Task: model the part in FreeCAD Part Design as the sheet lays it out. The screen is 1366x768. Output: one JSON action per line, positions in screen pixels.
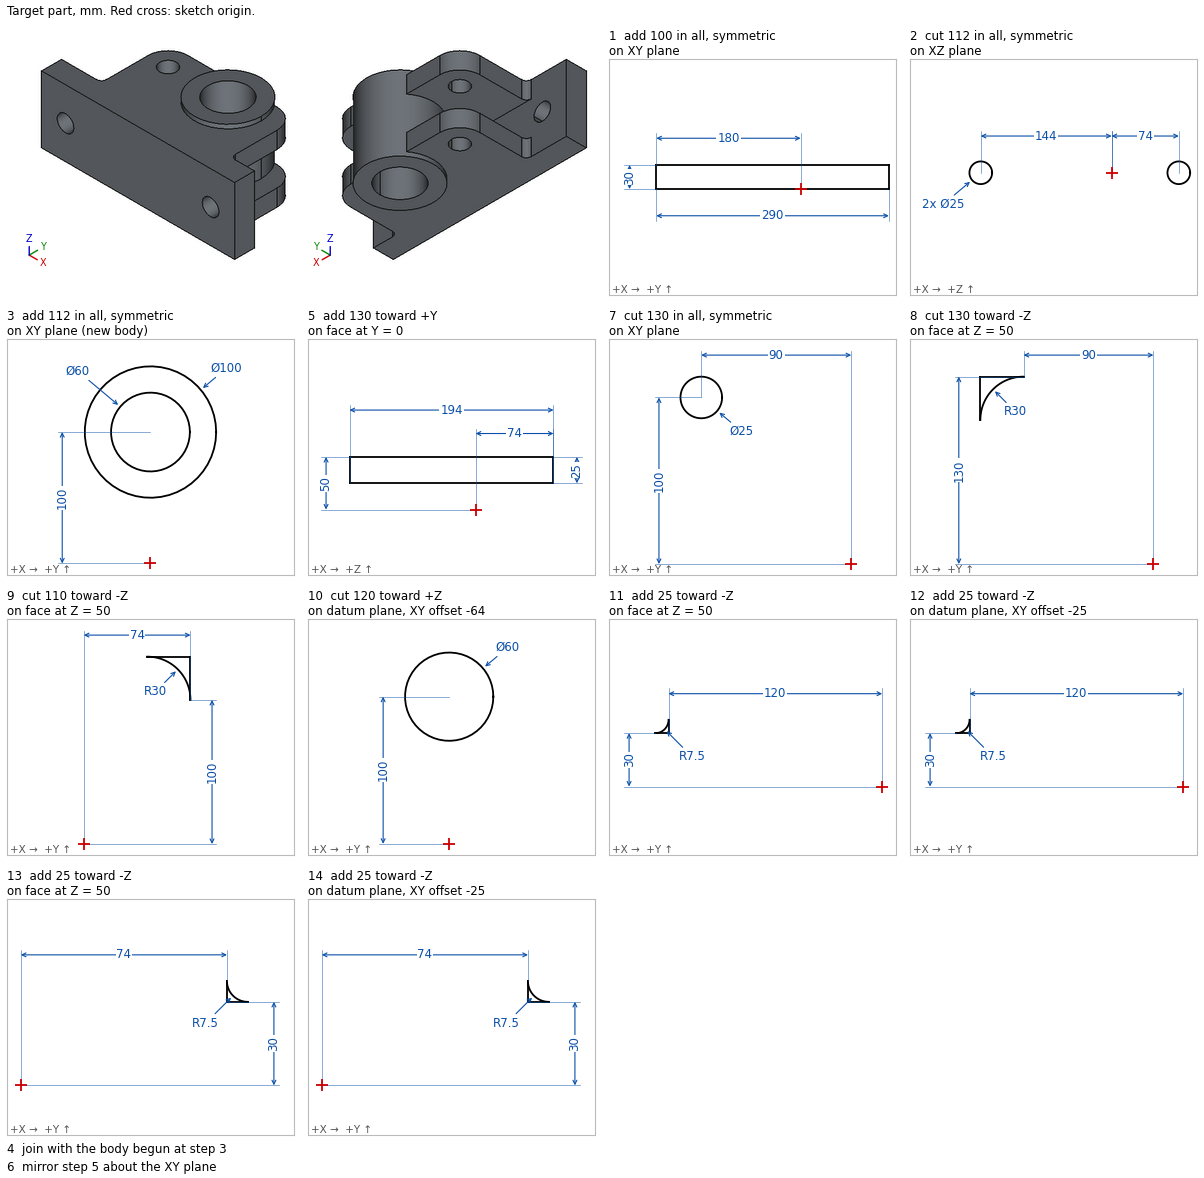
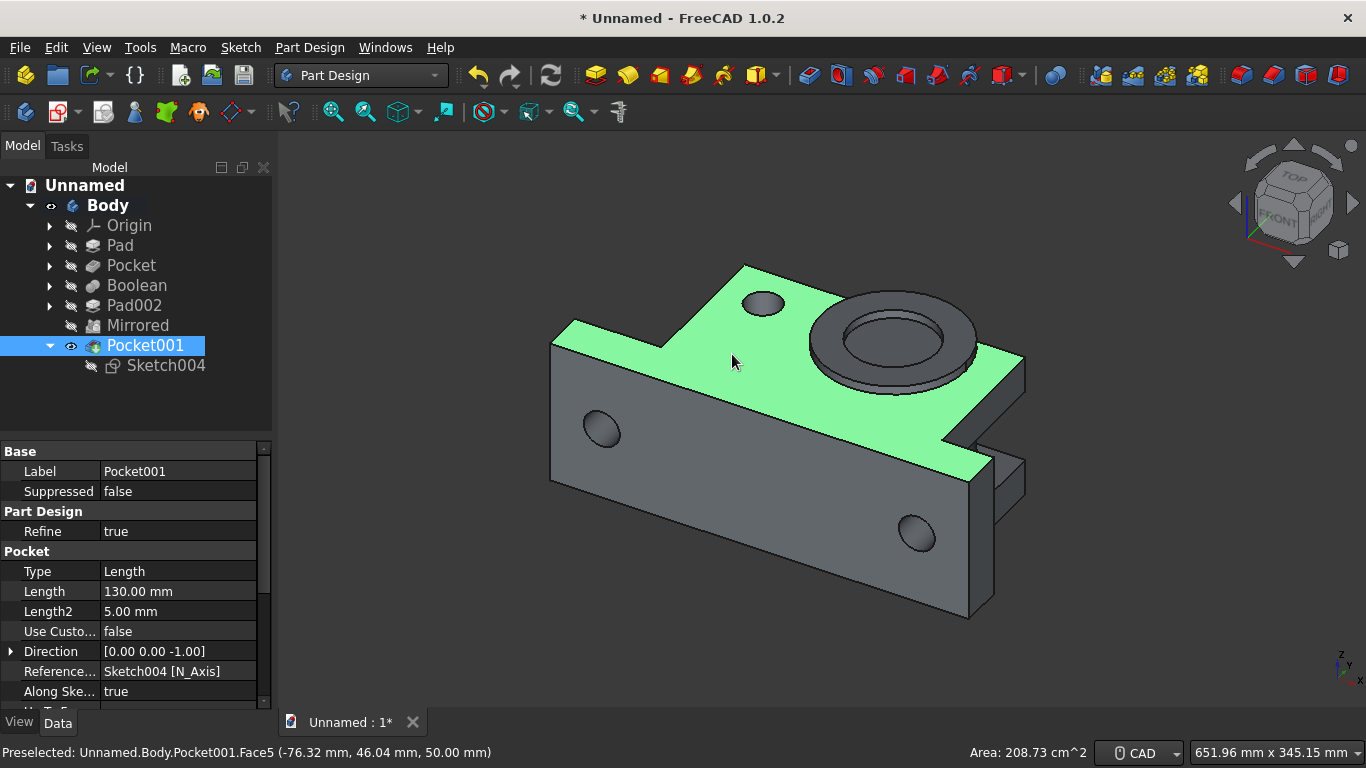
{"action": "left_click", "coordinate": [58, 112]}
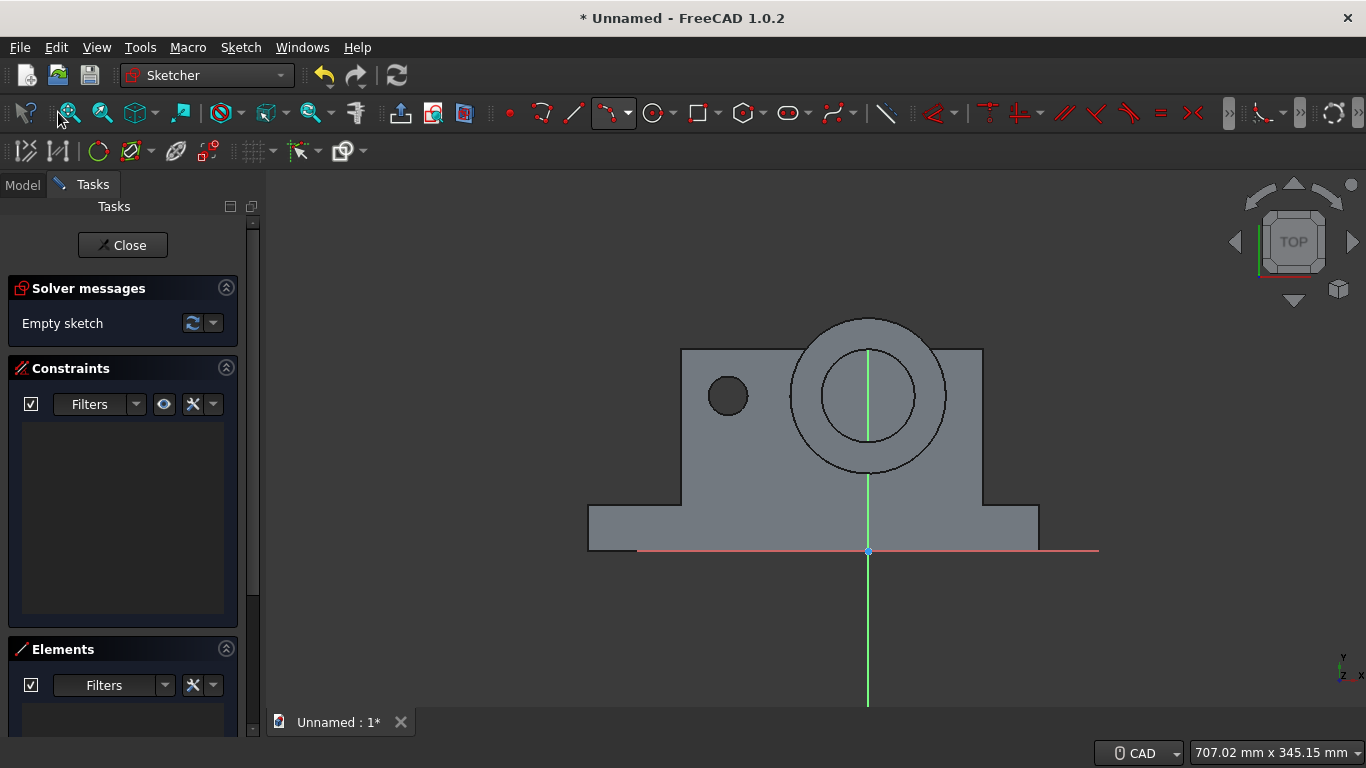
{"action": "scroll", "coordinate": [698, 362], "scroll_direction": "up", "scroll_amount": 10}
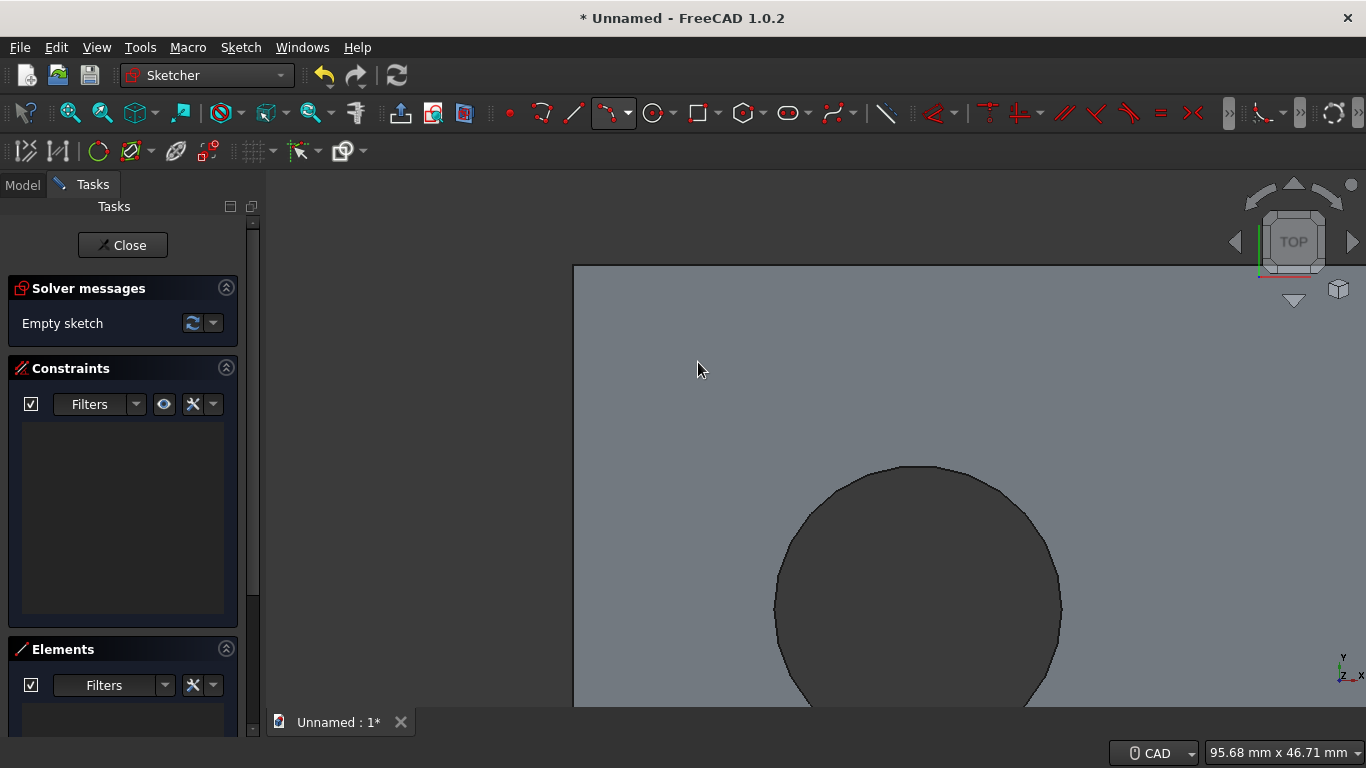
{"action": "left_click", "coordinate": [542, 114]}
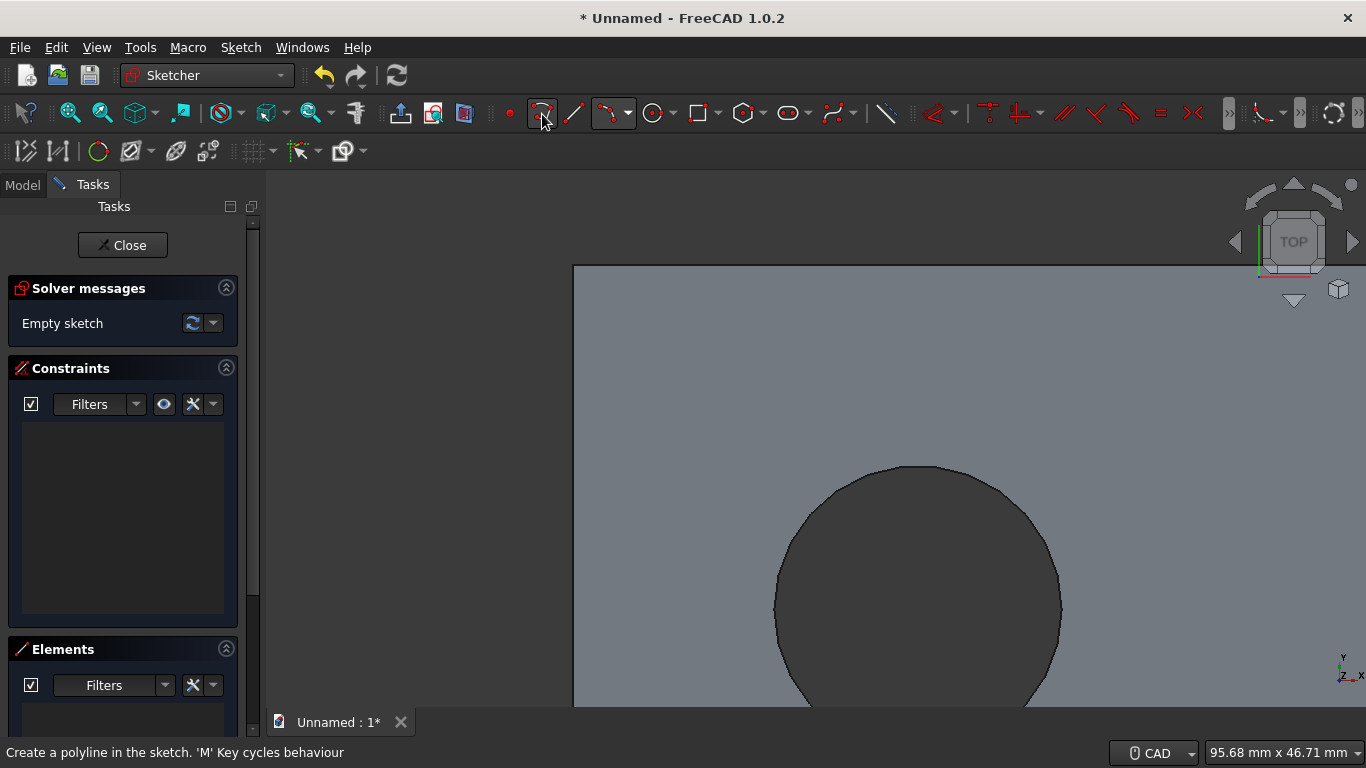
{"action": "left_click", "coordinate": [918, 265]}
{"action": "left_click", "coordinate": [573, 265]}
{"action": "left_click", "coordinate": [573, 610]}
{"action": "right_click", "coordinate": [573, 610]}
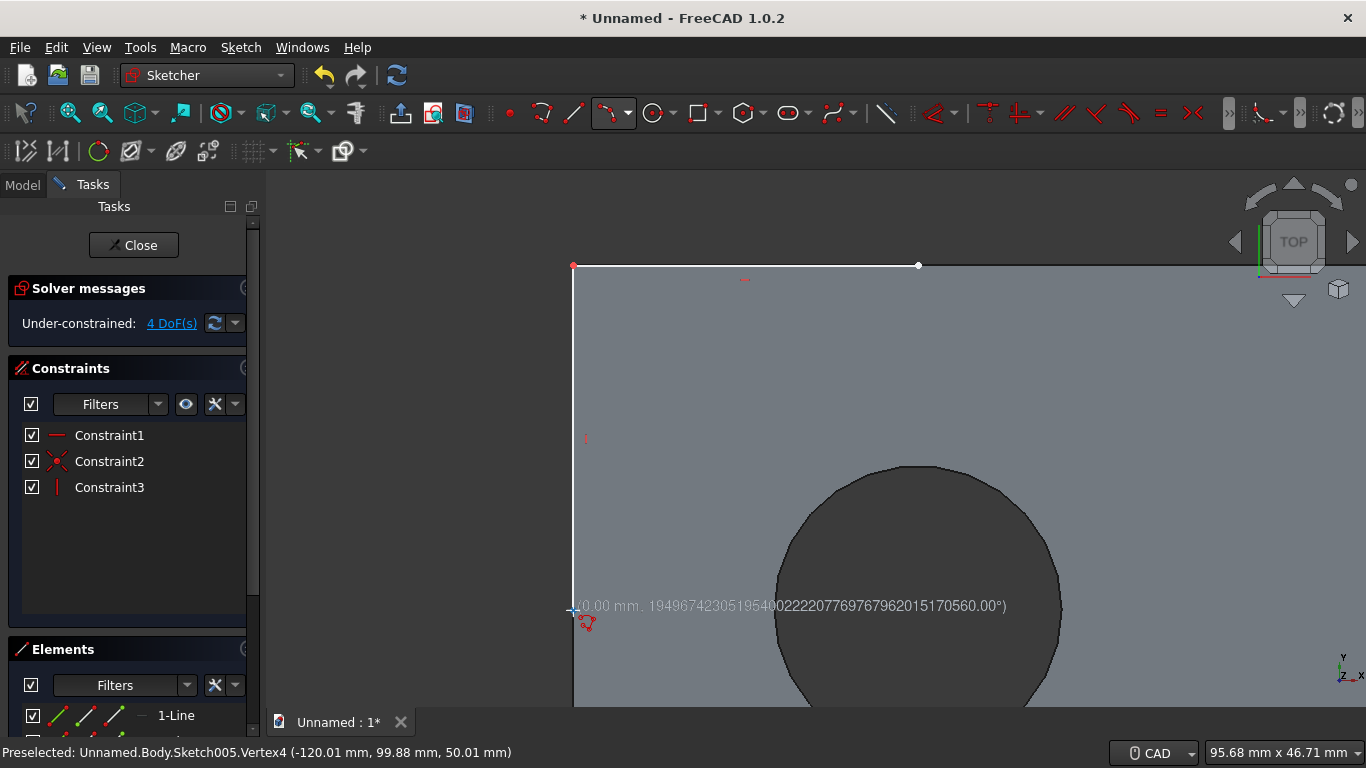
{"action": "left_click", "coordinate": [608, 114]}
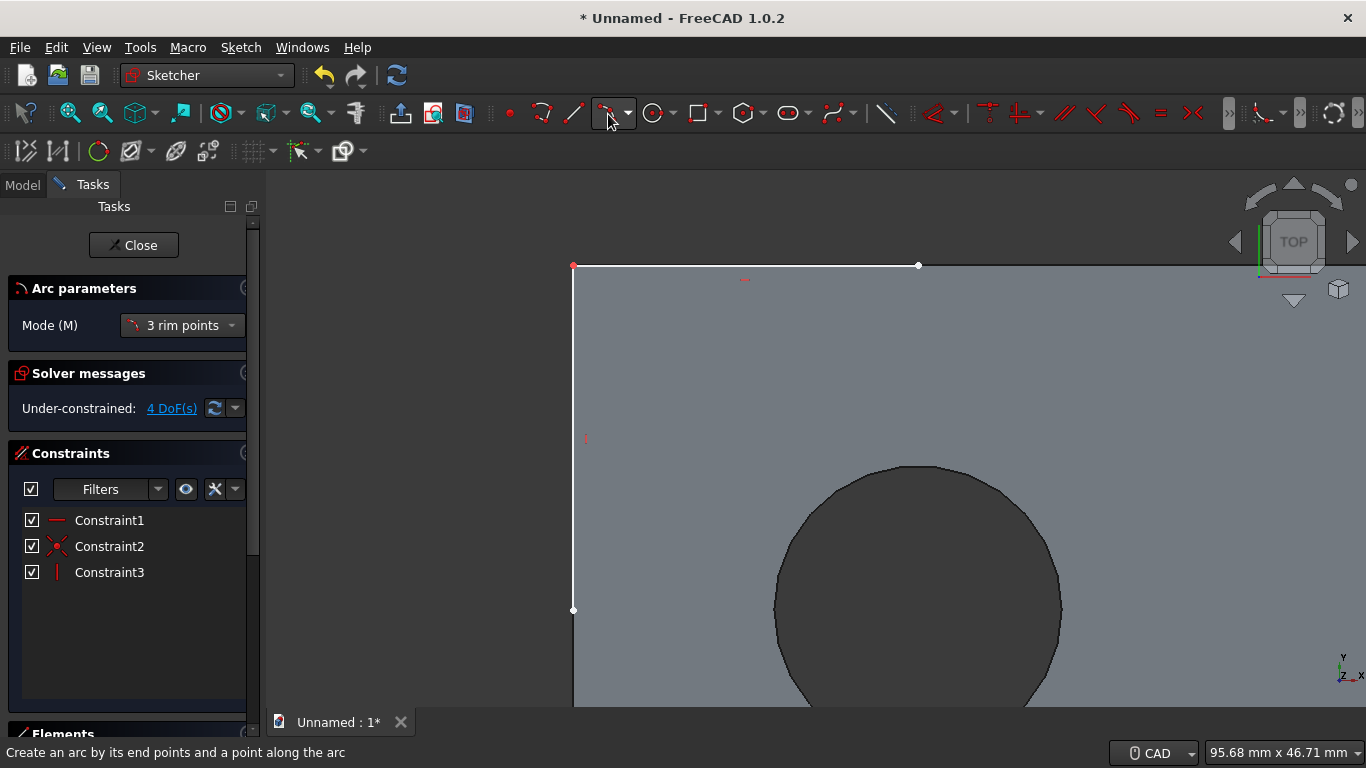
{"action": "left_click", "coordinate": [573, 611]}
{"action": "left_click", "coordinate": [918, 266]}
{"action": "left_click", "coordinate": [674, 366]}
{"action": "key", "text": "Escape"}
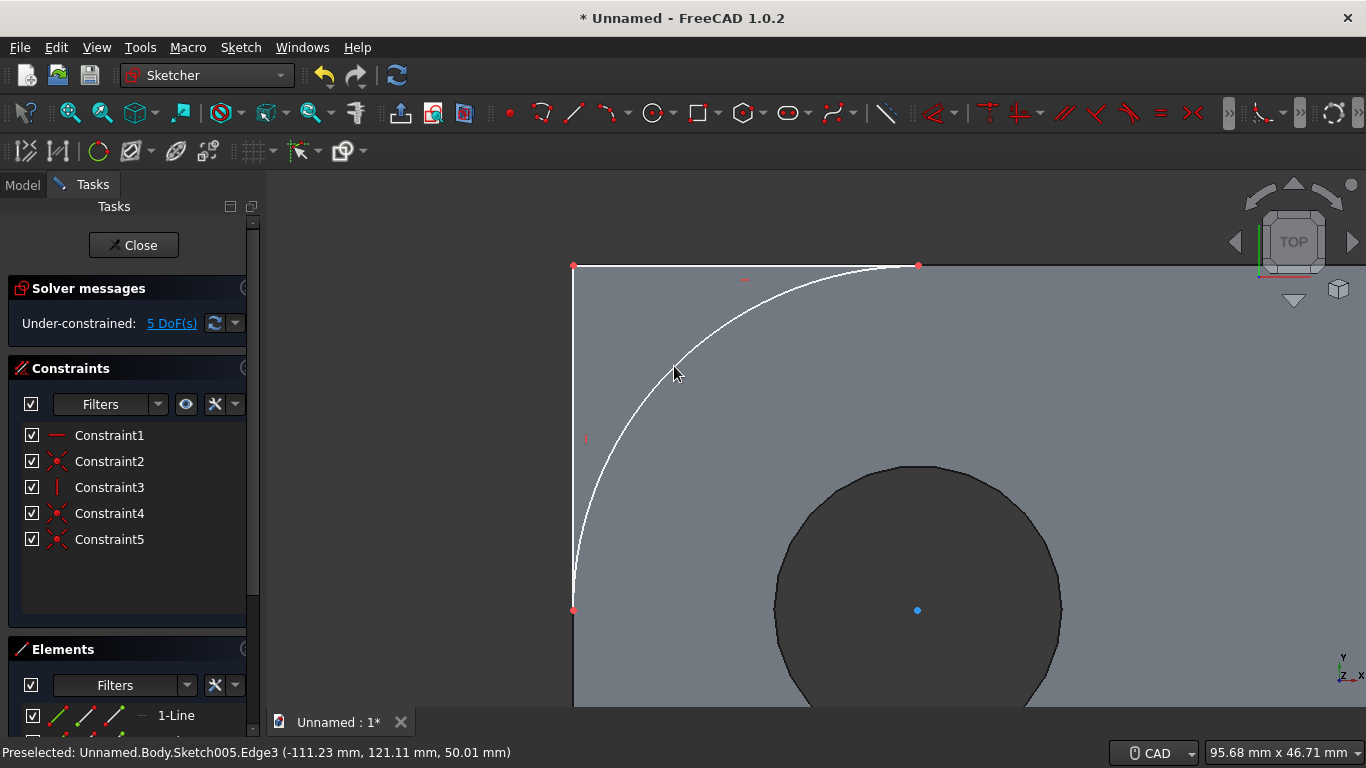
{"action": "left_click", "coordinate": [815, 266]}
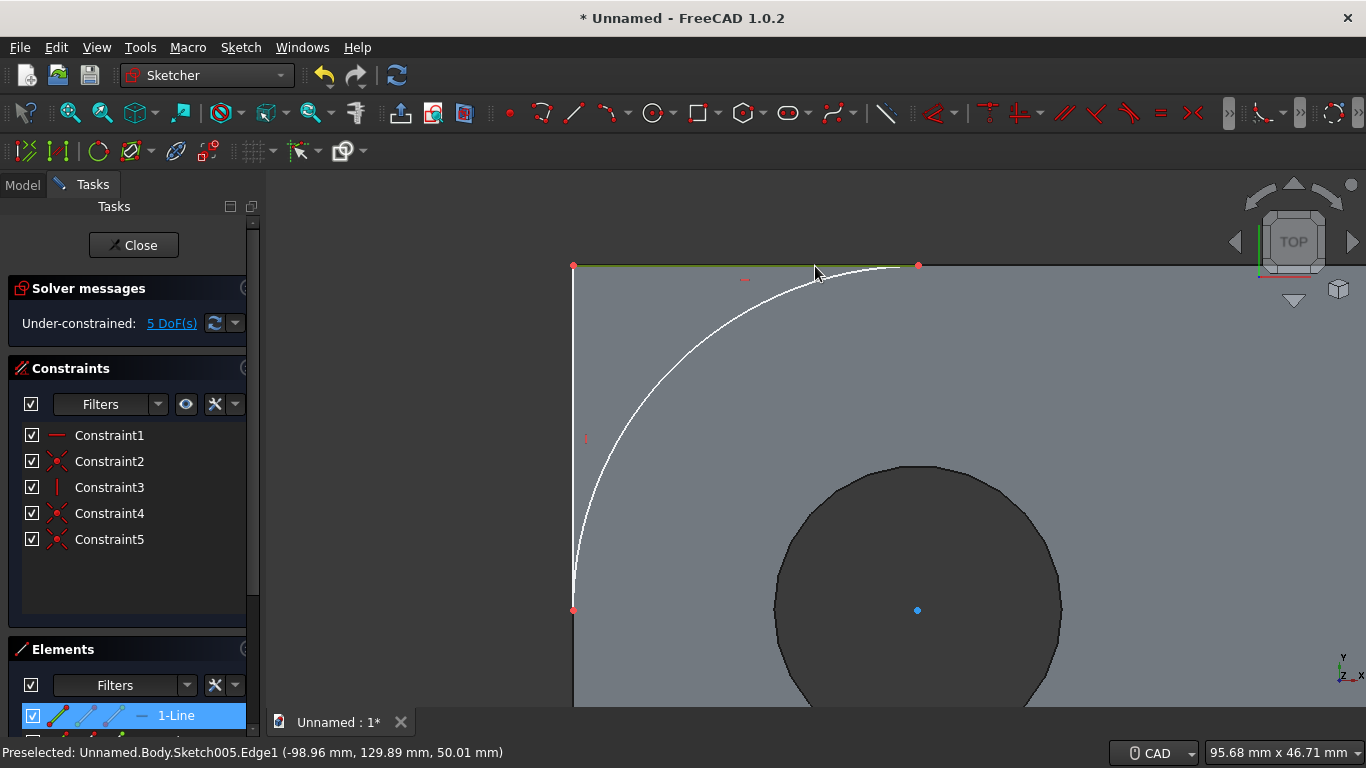
{"action": "left_click", "coordinate": [761, 304]}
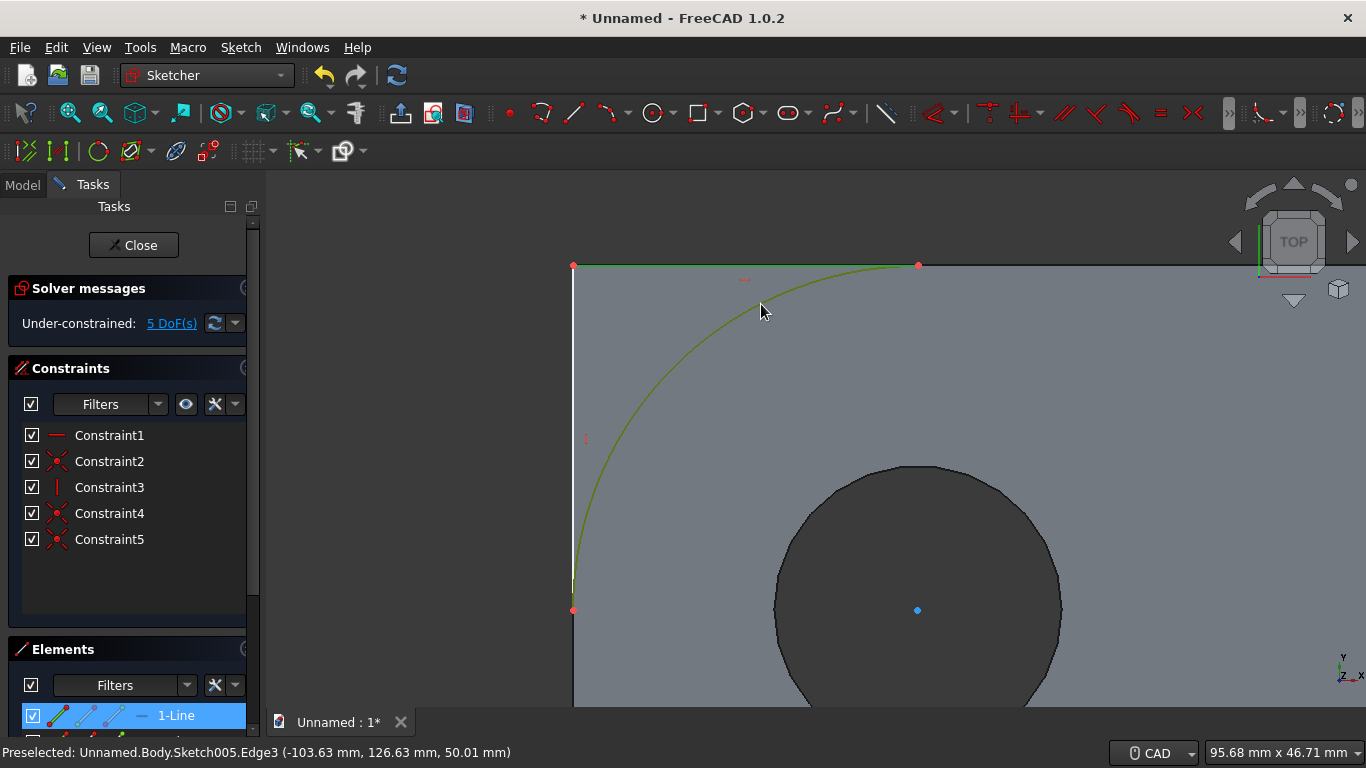
{"action": "left_click", "coordinate": [1130, 114]}